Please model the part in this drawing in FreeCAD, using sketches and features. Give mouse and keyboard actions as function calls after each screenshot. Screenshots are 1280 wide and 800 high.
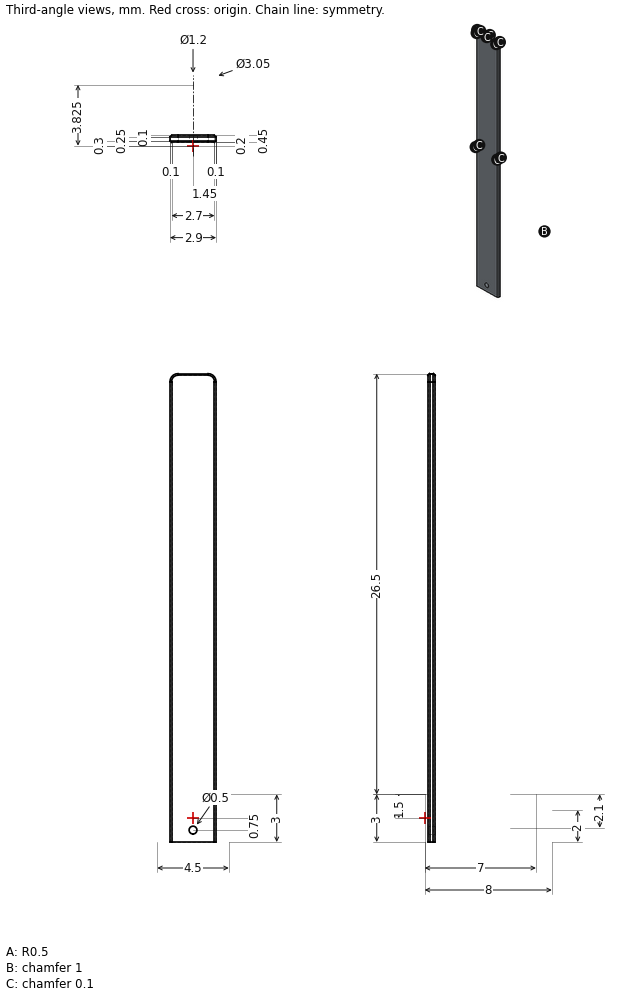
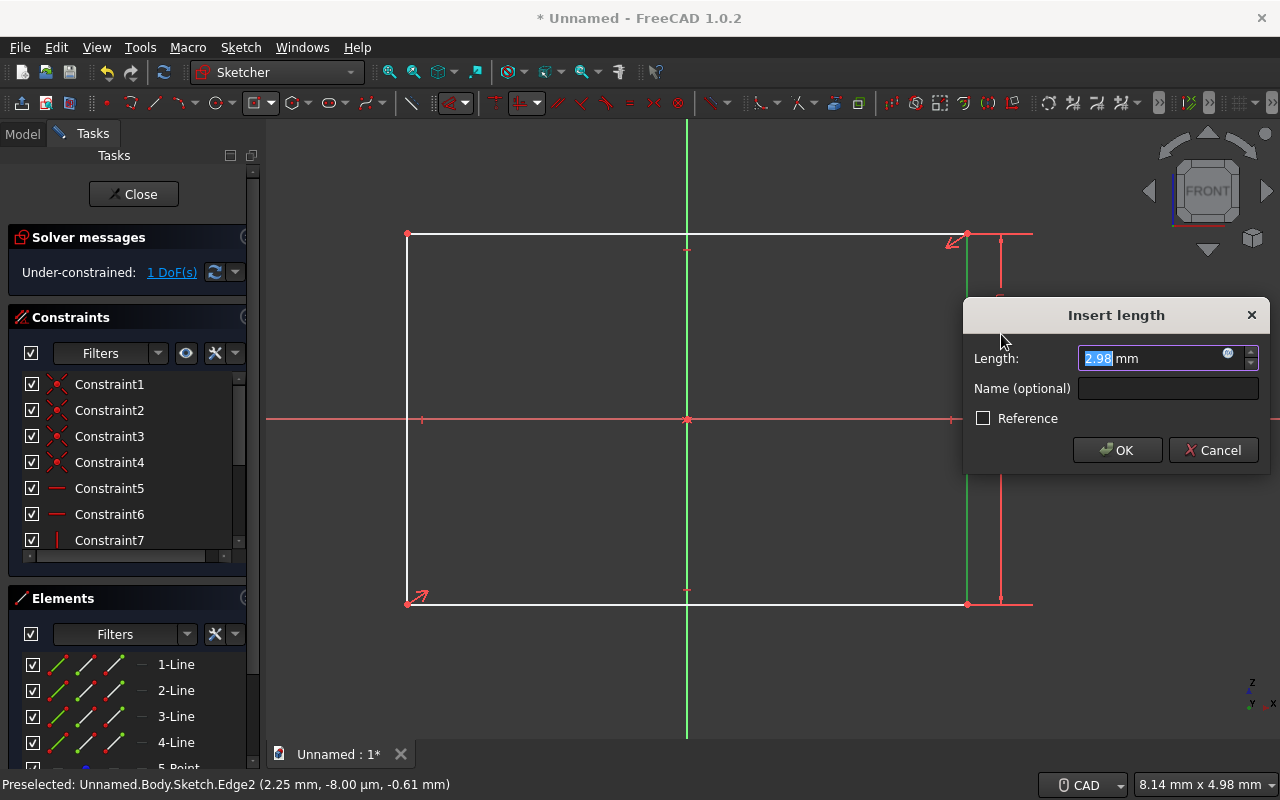
text(3)
key(Return)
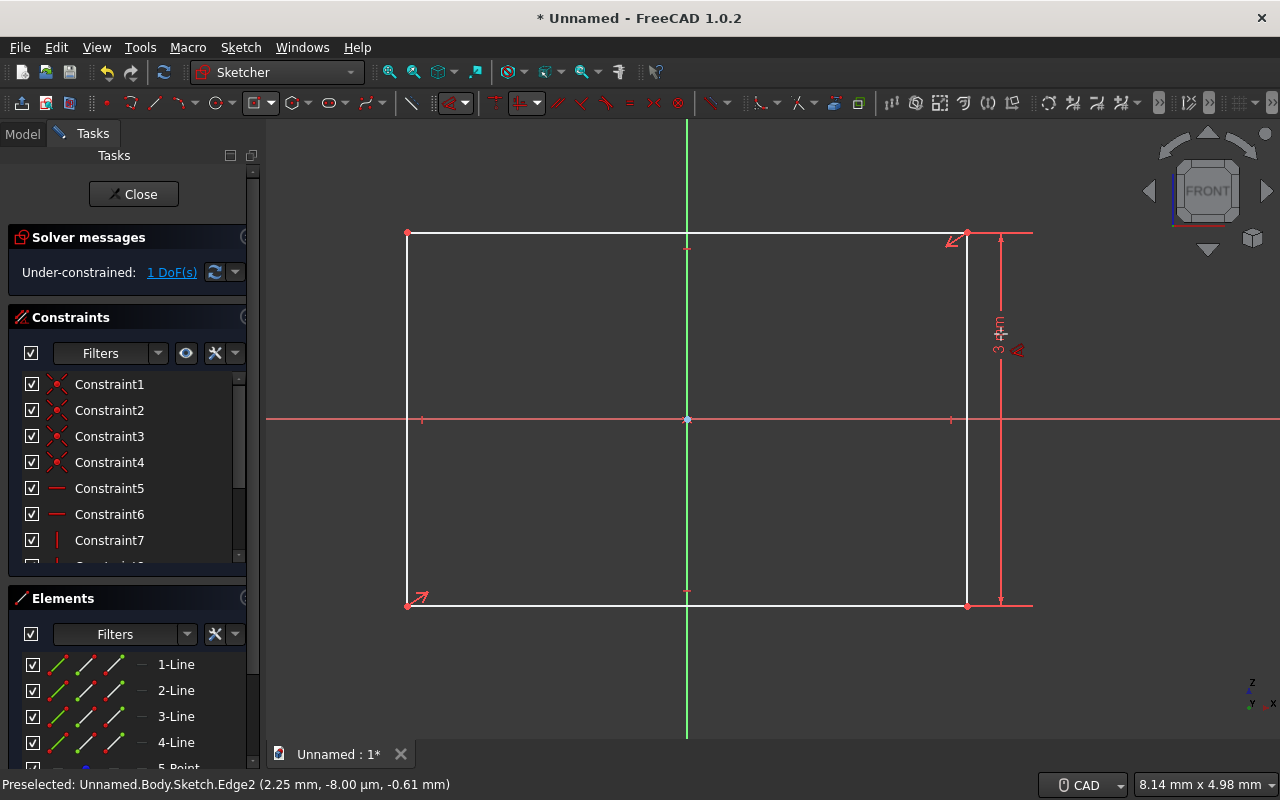
click(575, 606)
click(558, 640)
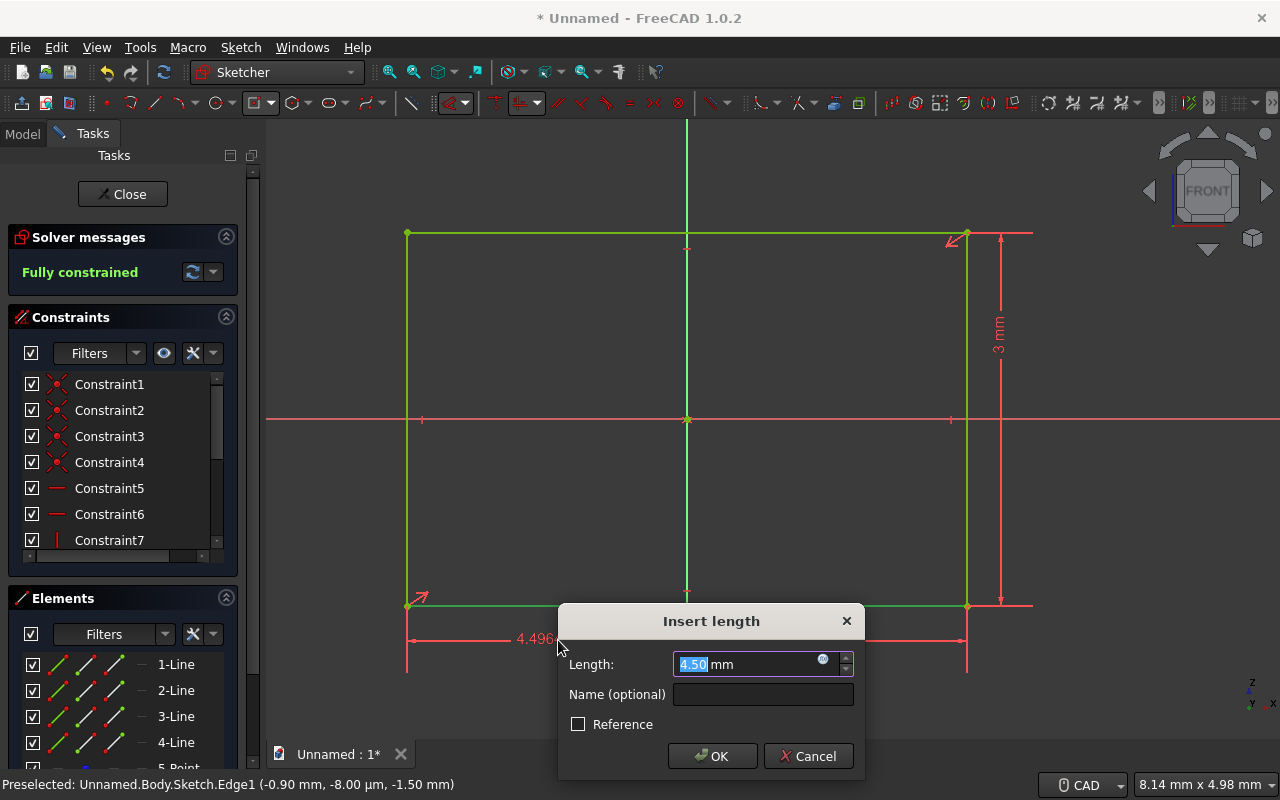
text(4.5)
key(Return)
key(Escape)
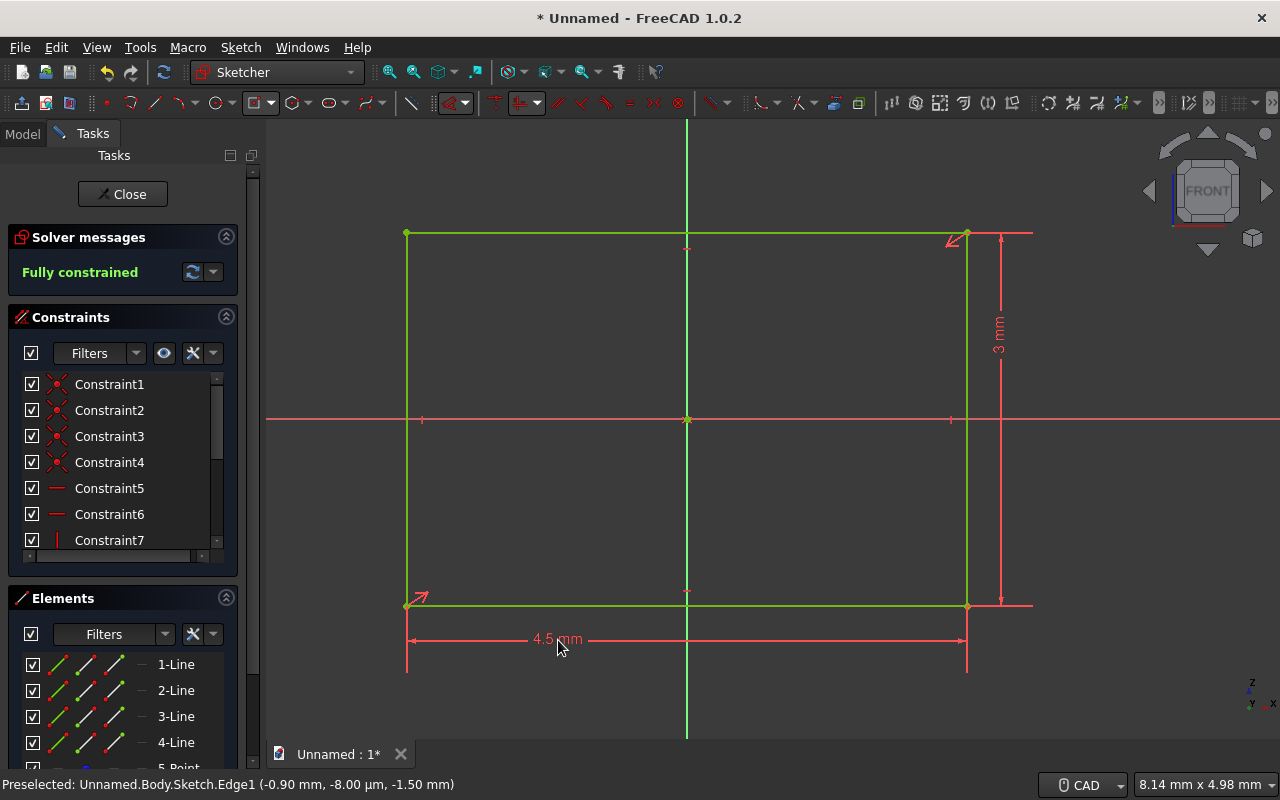
click(123, 194)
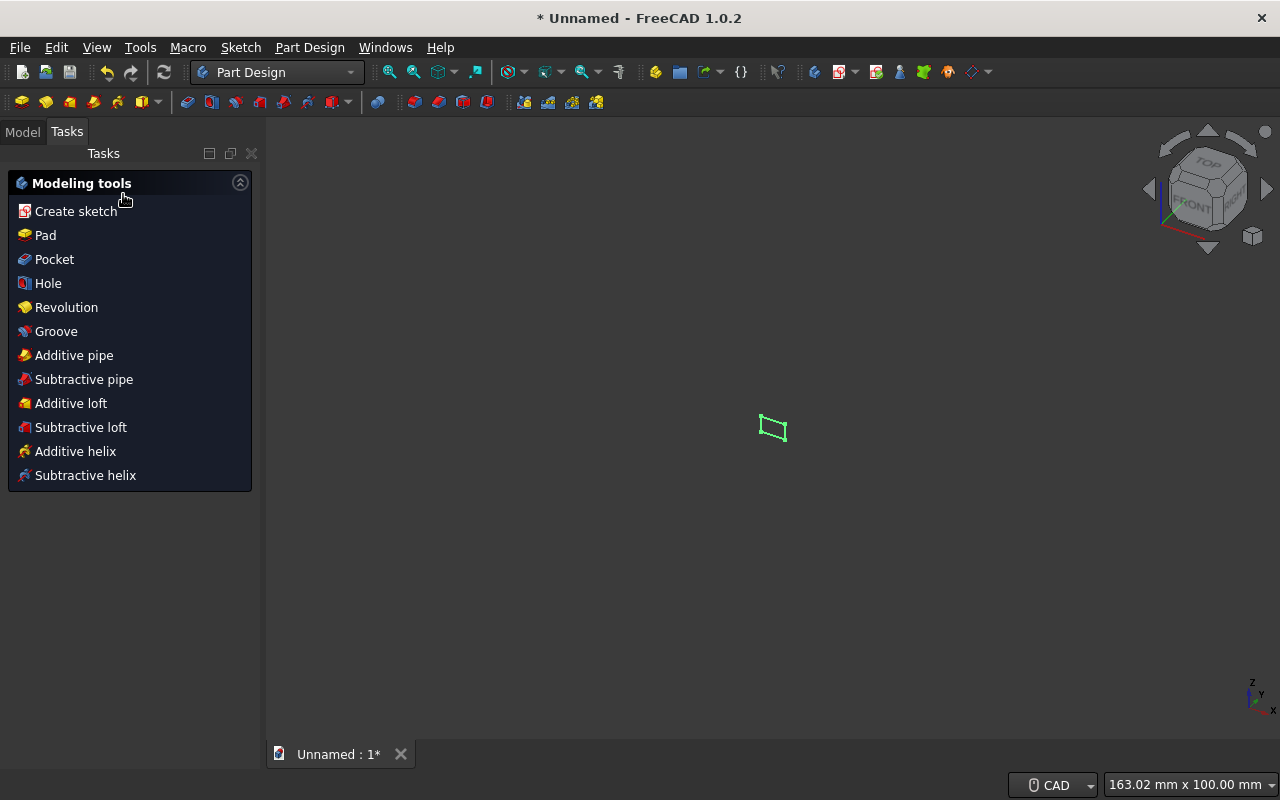
click(22, 102)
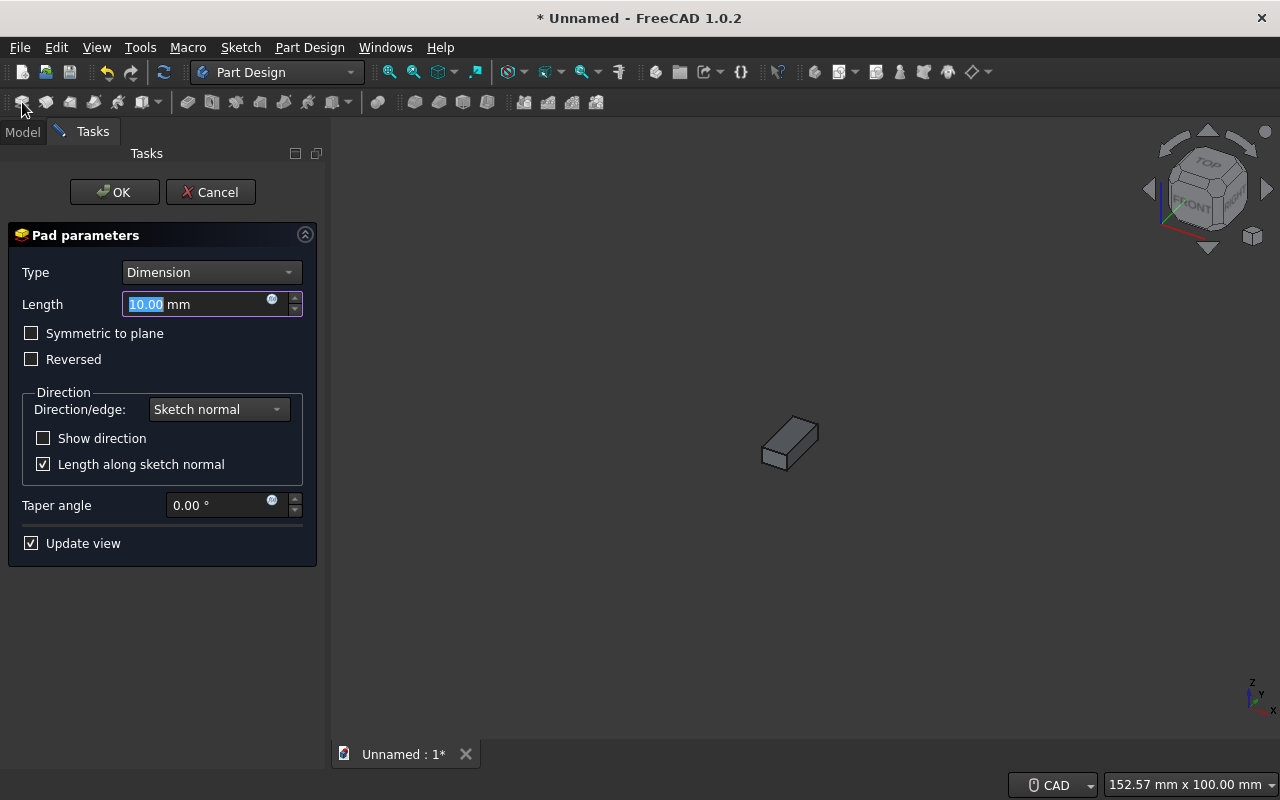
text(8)
key(Tab)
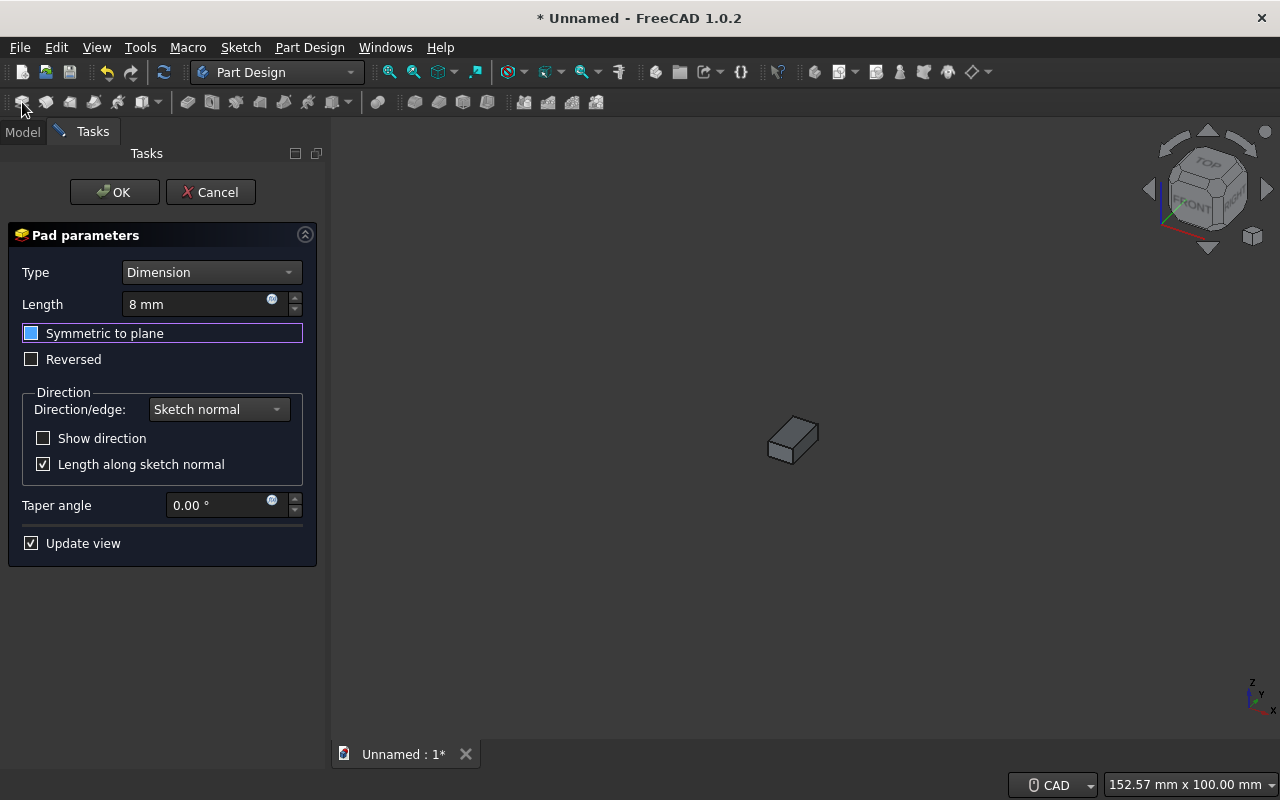
click(30, 359)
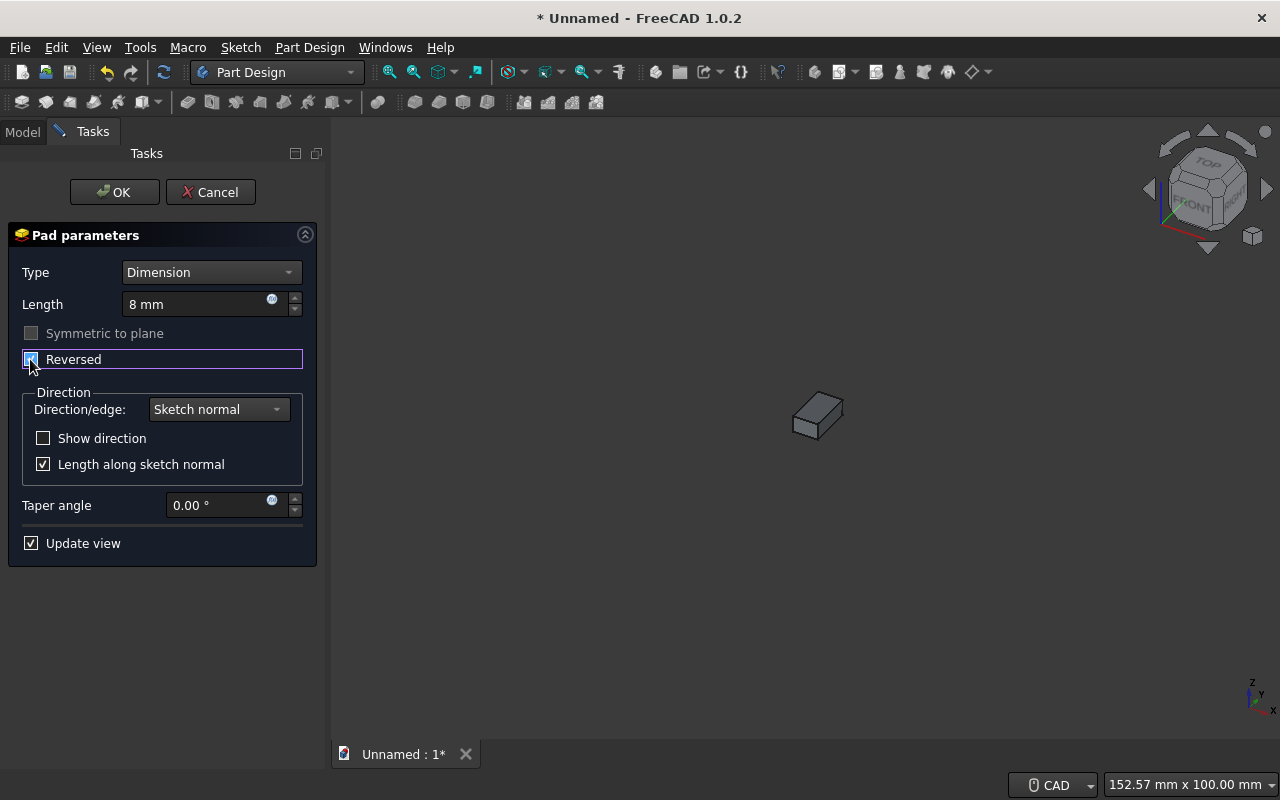
click(115, 192)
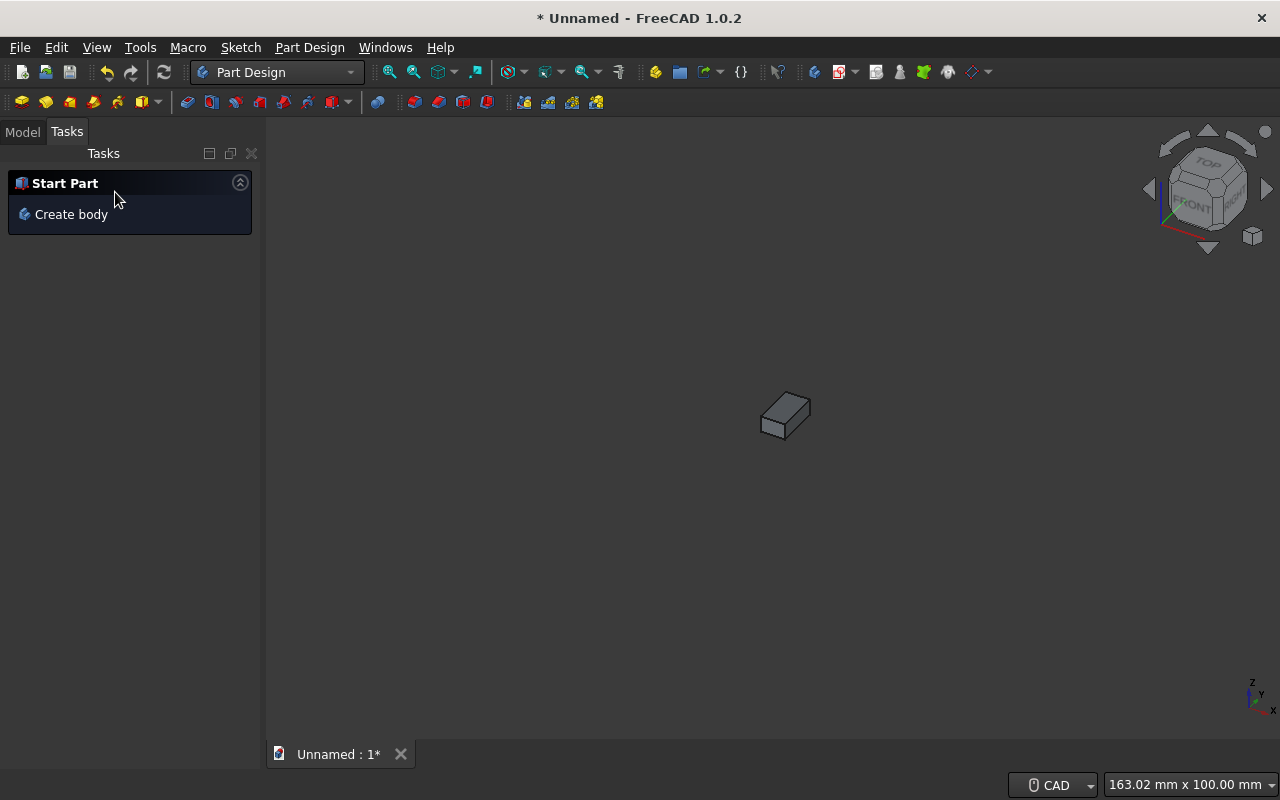
click(390, 72)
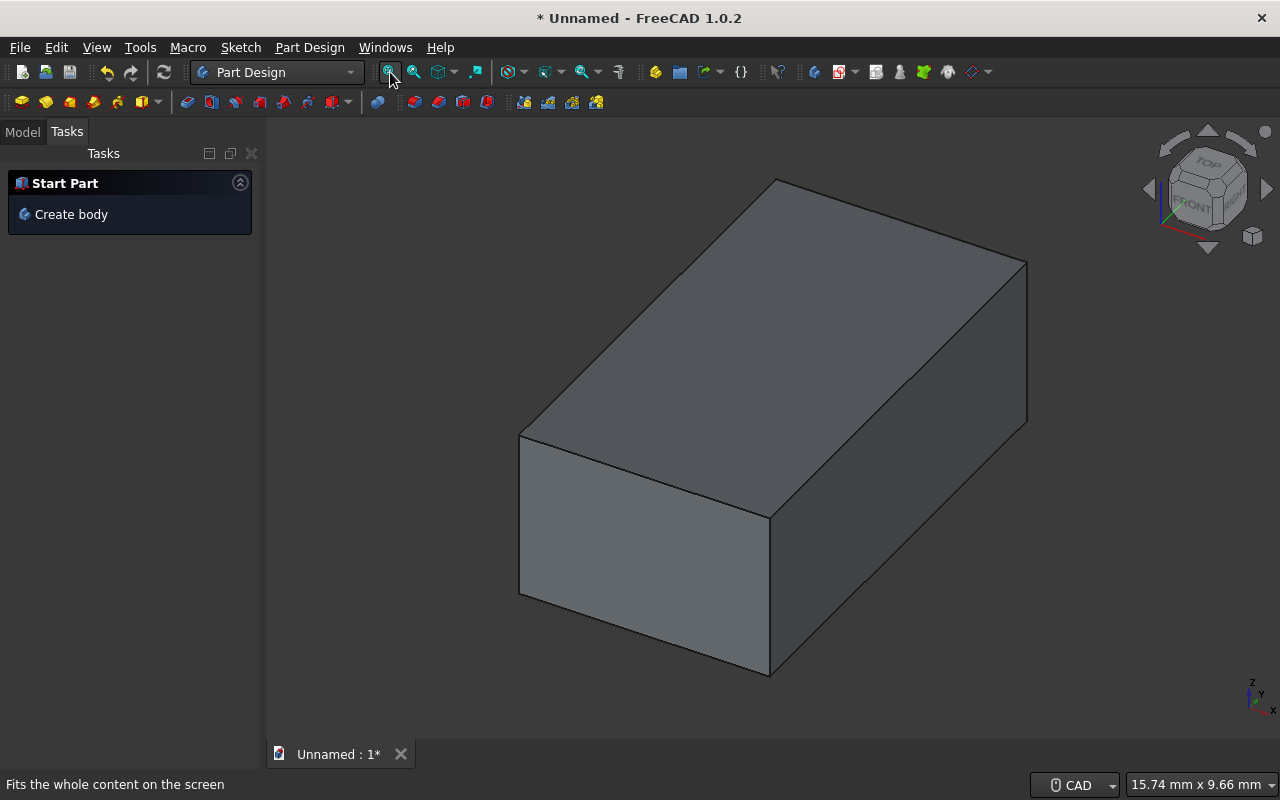
click(810, 311)